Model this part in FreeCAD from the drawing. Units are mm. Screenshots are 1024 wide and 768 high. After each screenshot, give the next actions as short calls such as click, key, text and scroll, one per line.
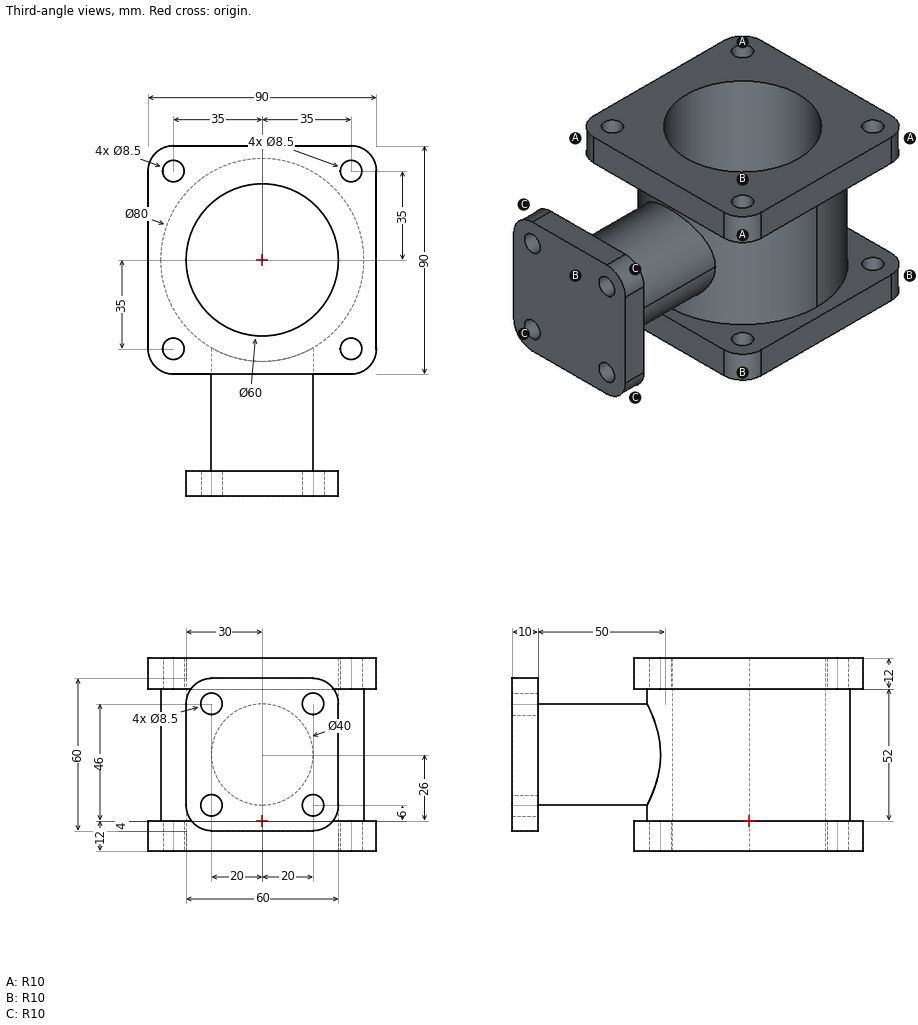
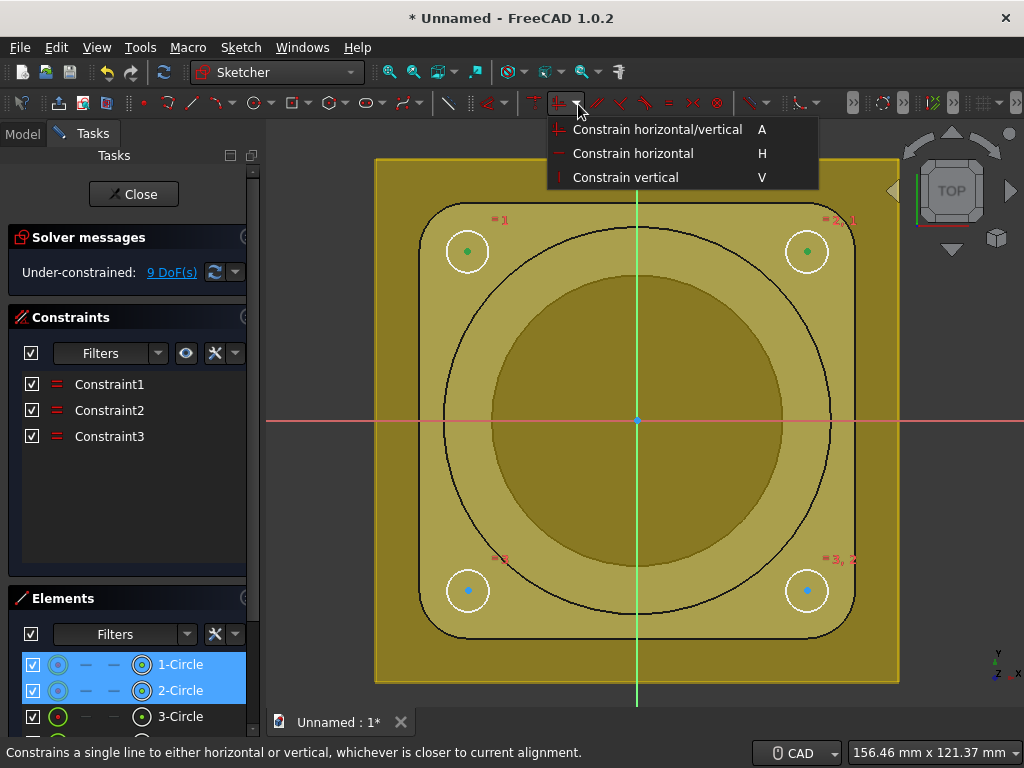
click(683, 153)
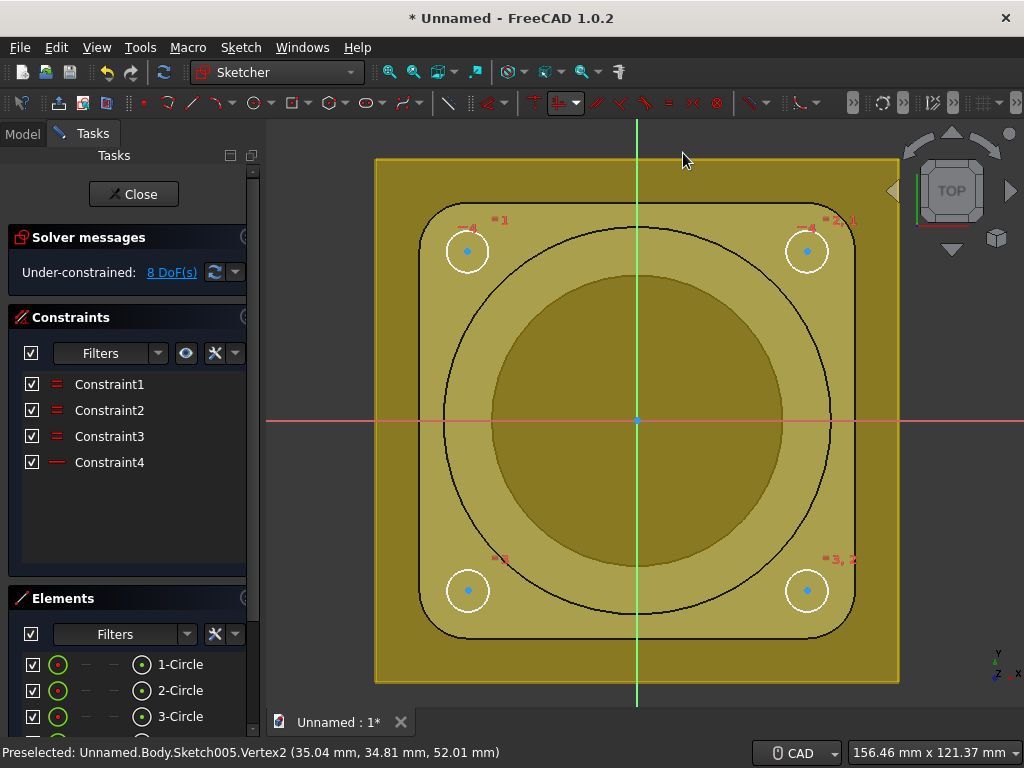
click(807, 252)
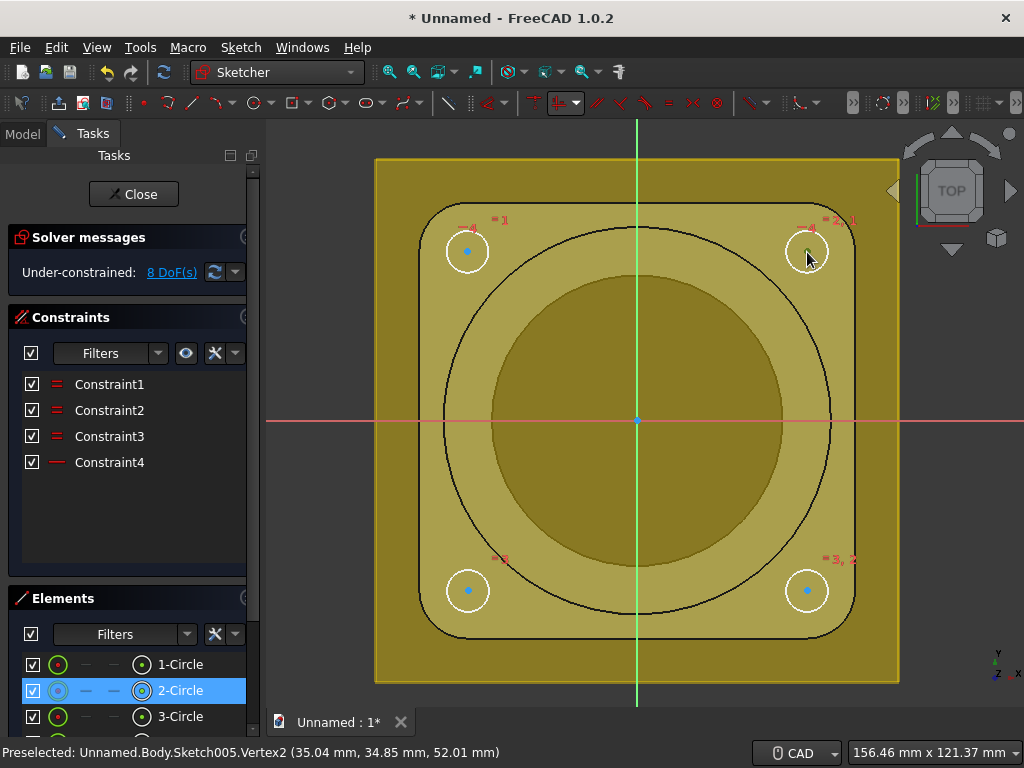
click(807, 591)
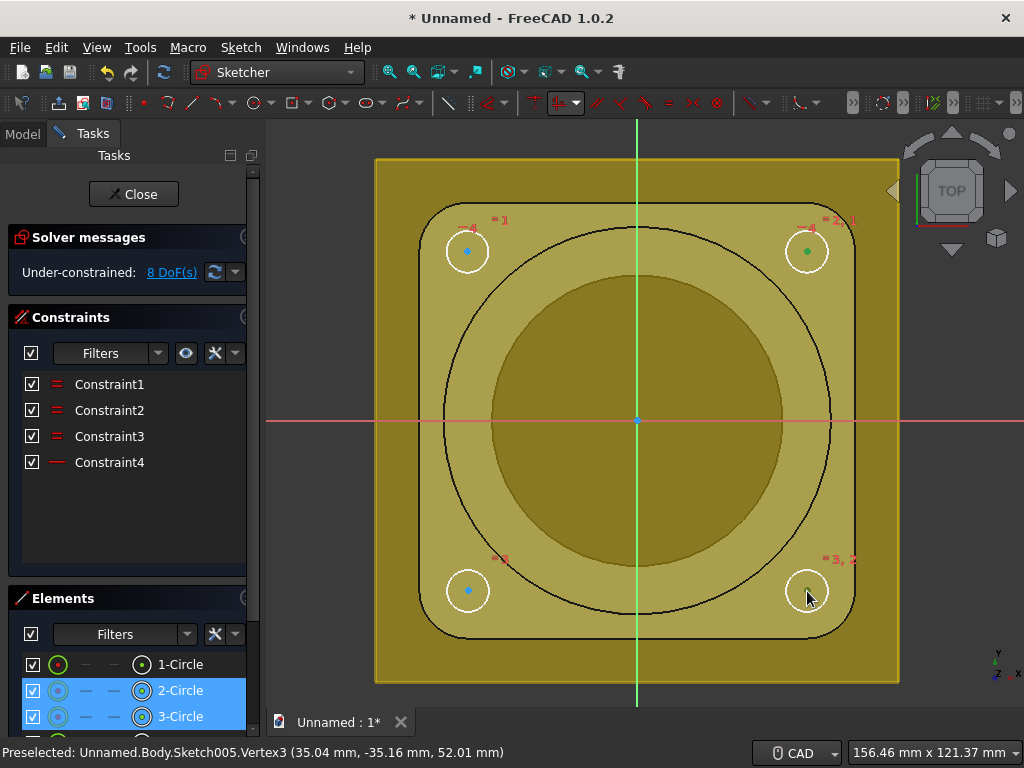
click(578, 104)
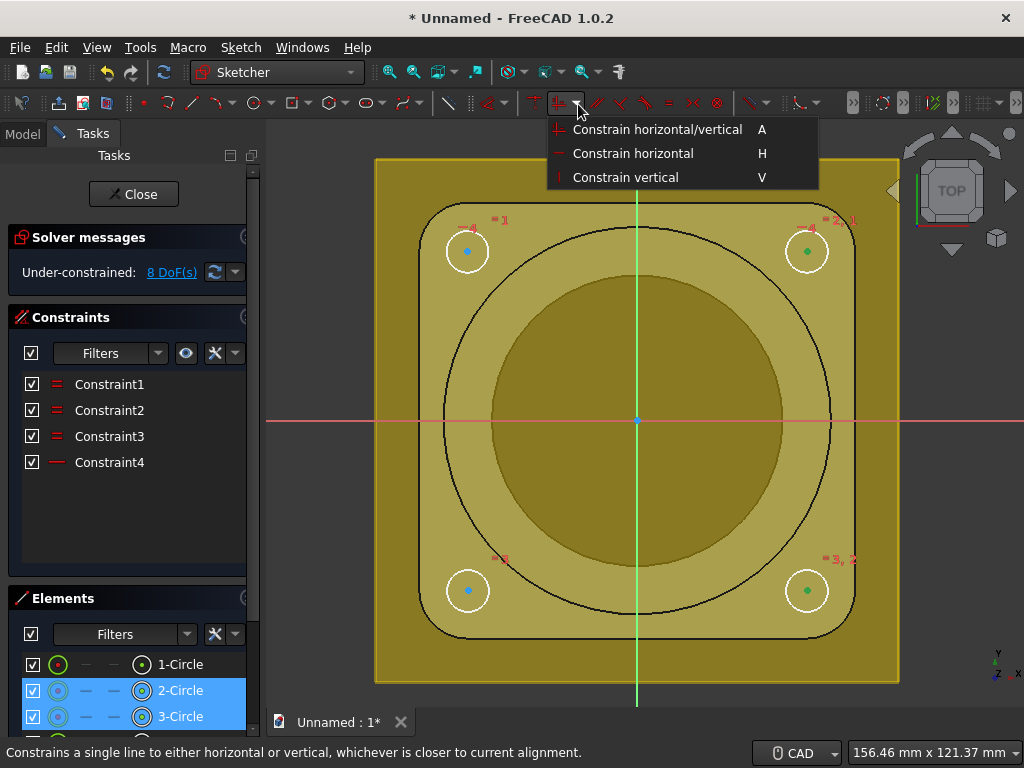
click(683, 177)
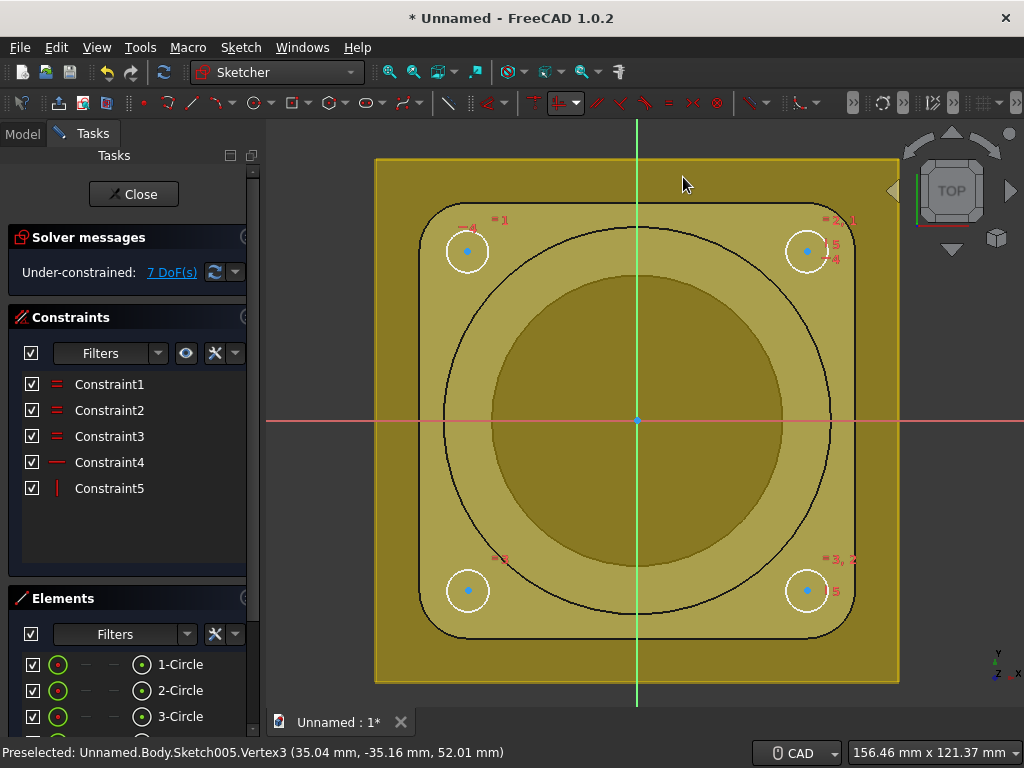
click(468, 252)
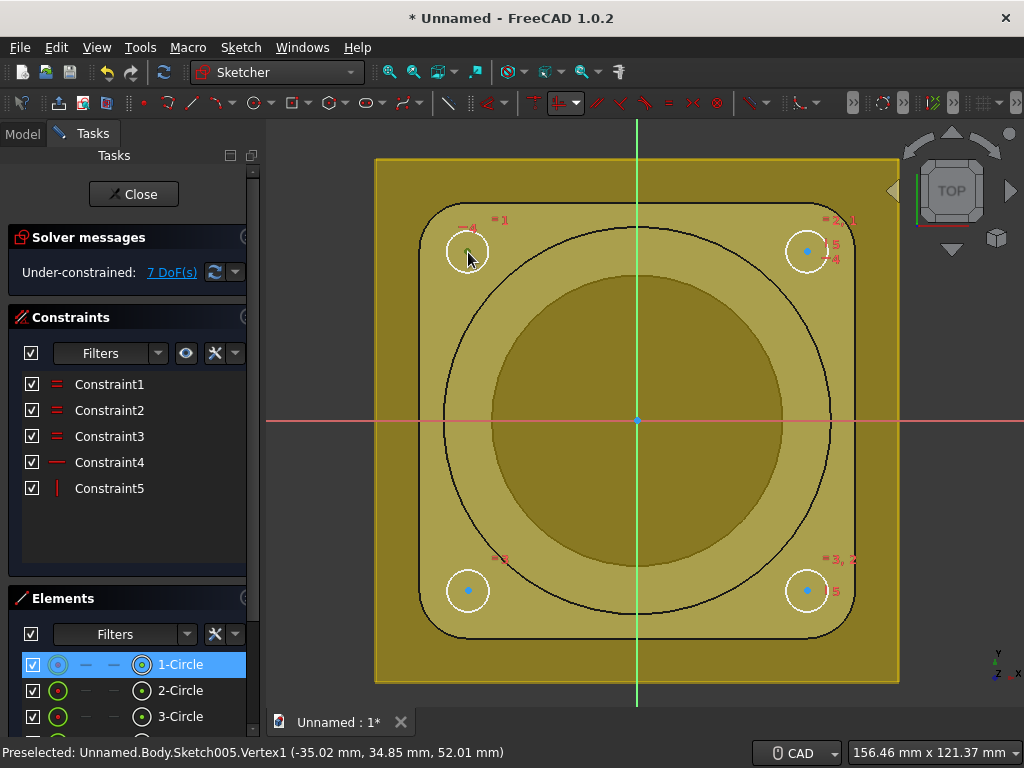
click(468, 591)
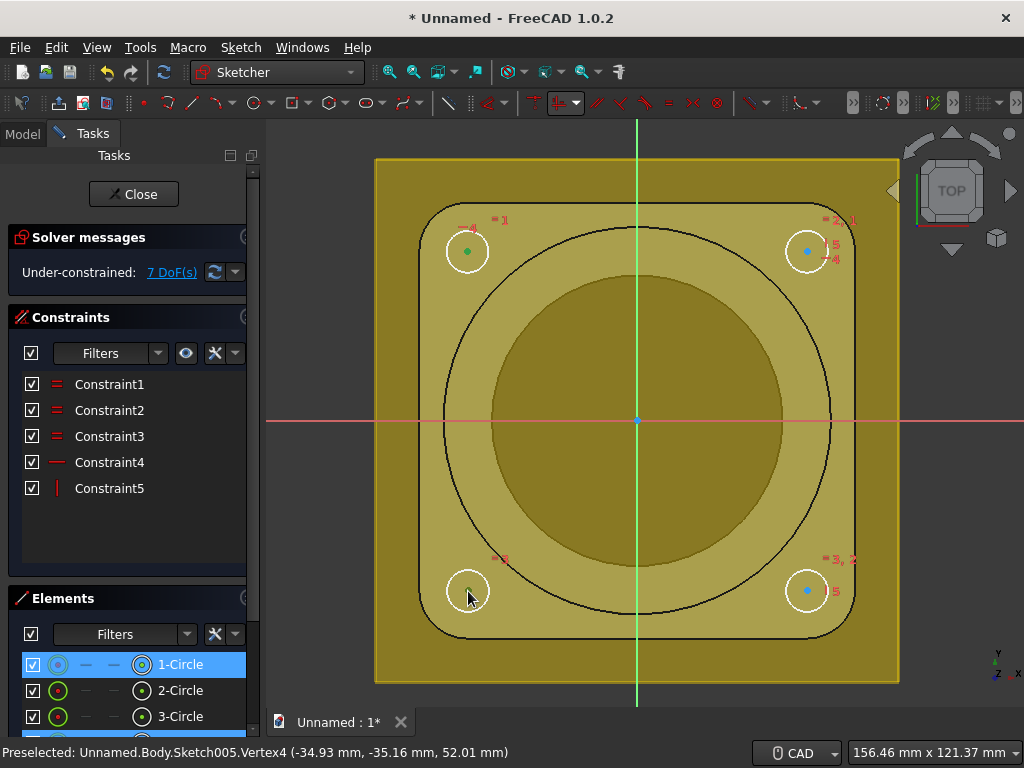
key(v)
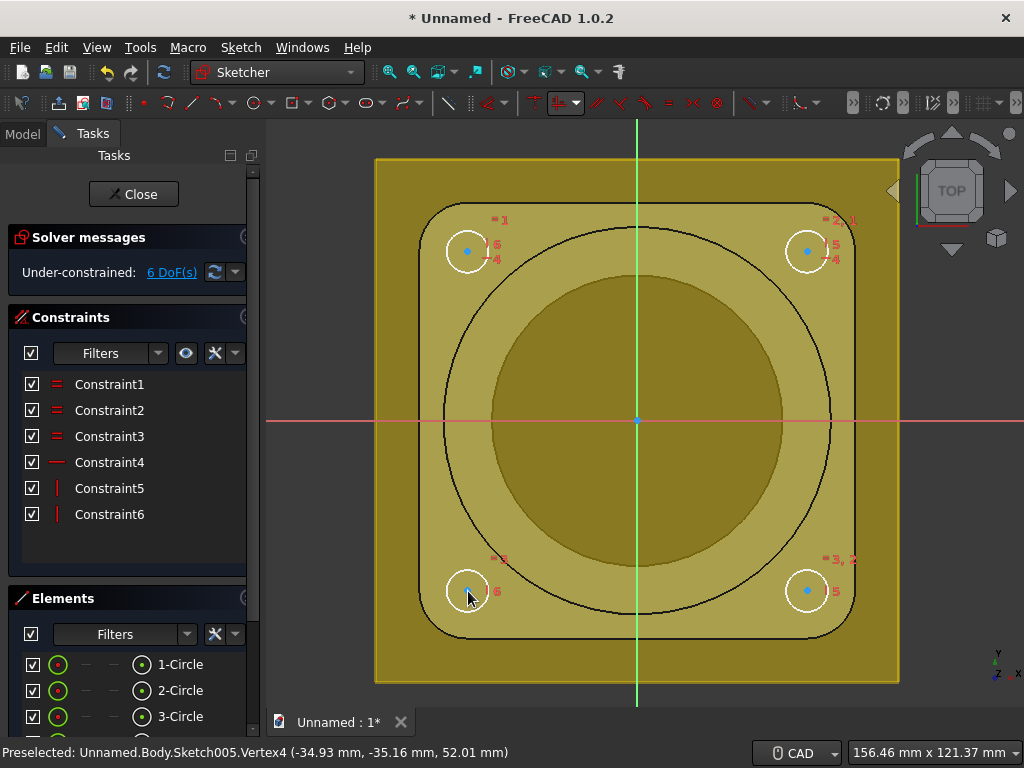
click(807, 591)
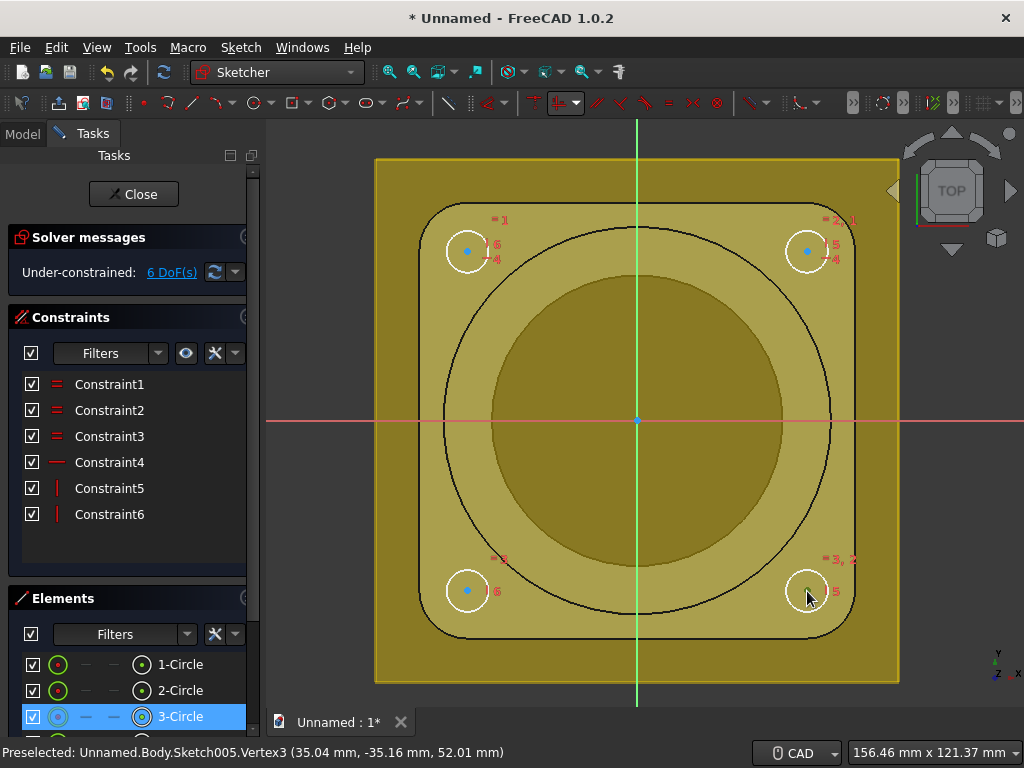
click(468, 591)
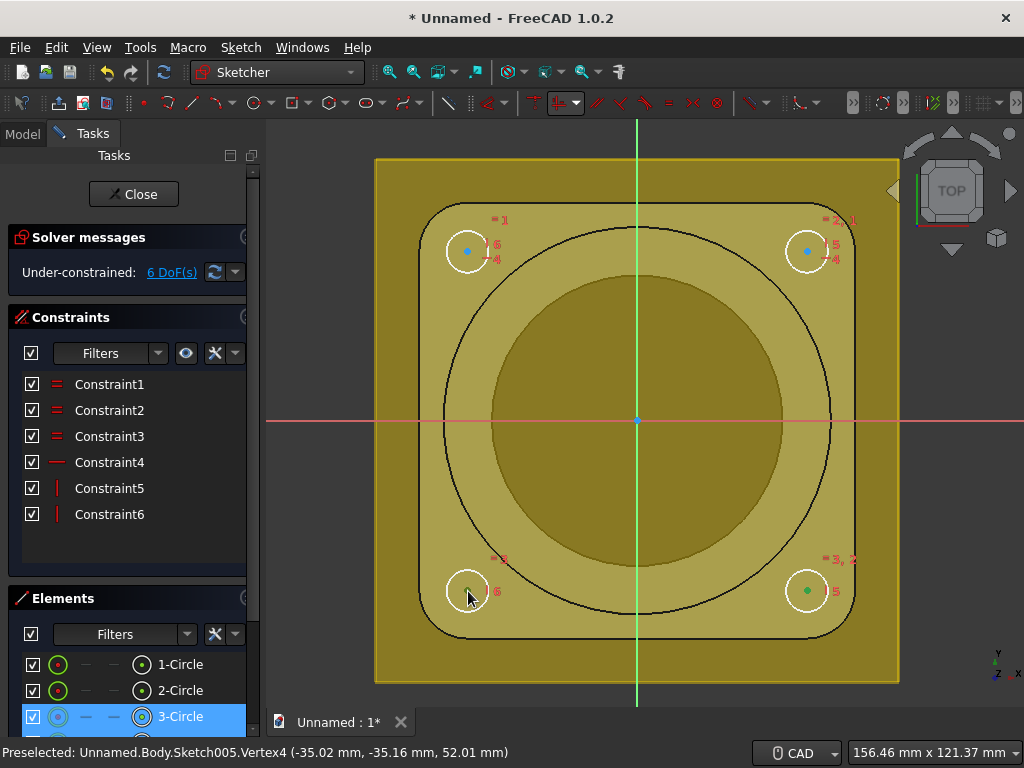
click(578, 104)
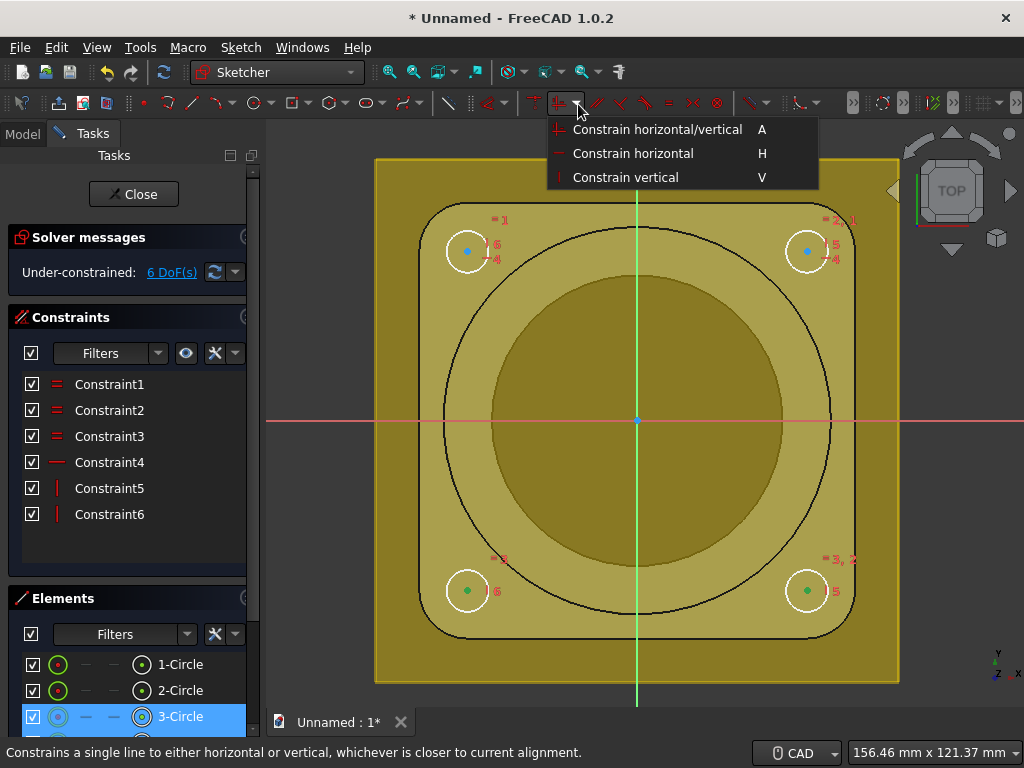
click(683, 153)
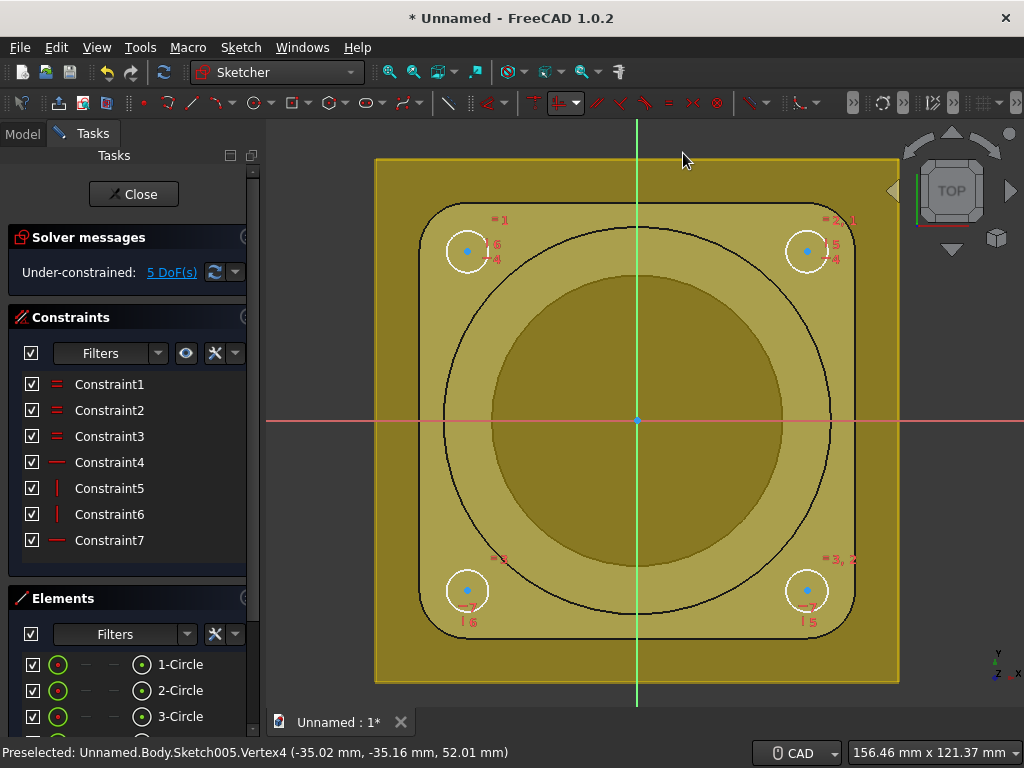
click(488, 104)